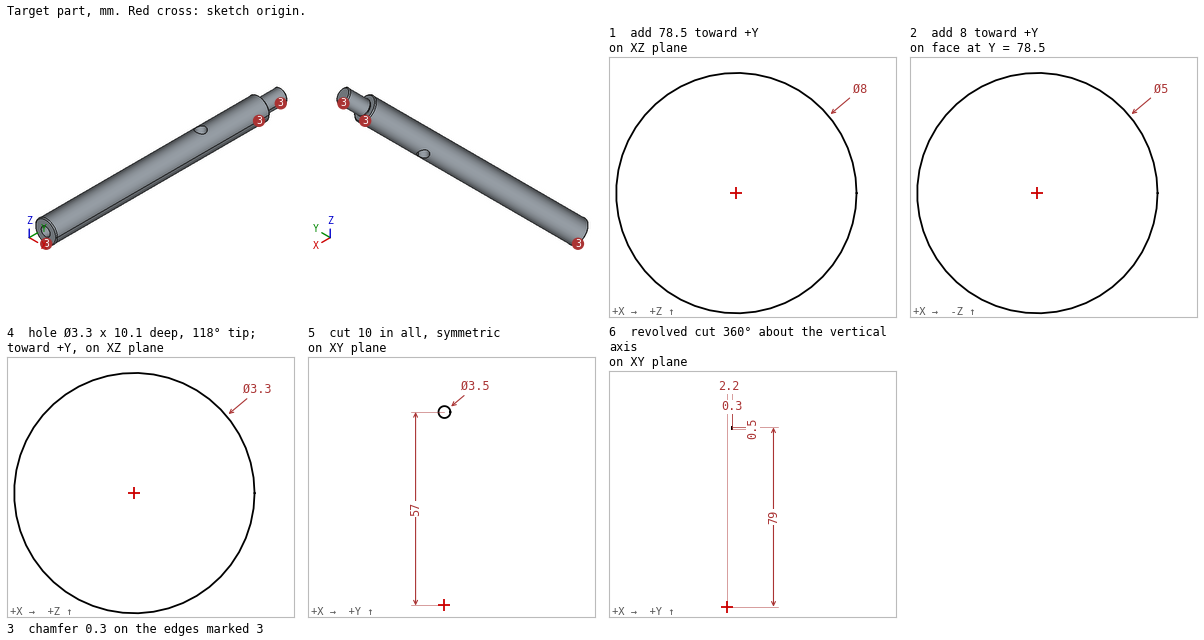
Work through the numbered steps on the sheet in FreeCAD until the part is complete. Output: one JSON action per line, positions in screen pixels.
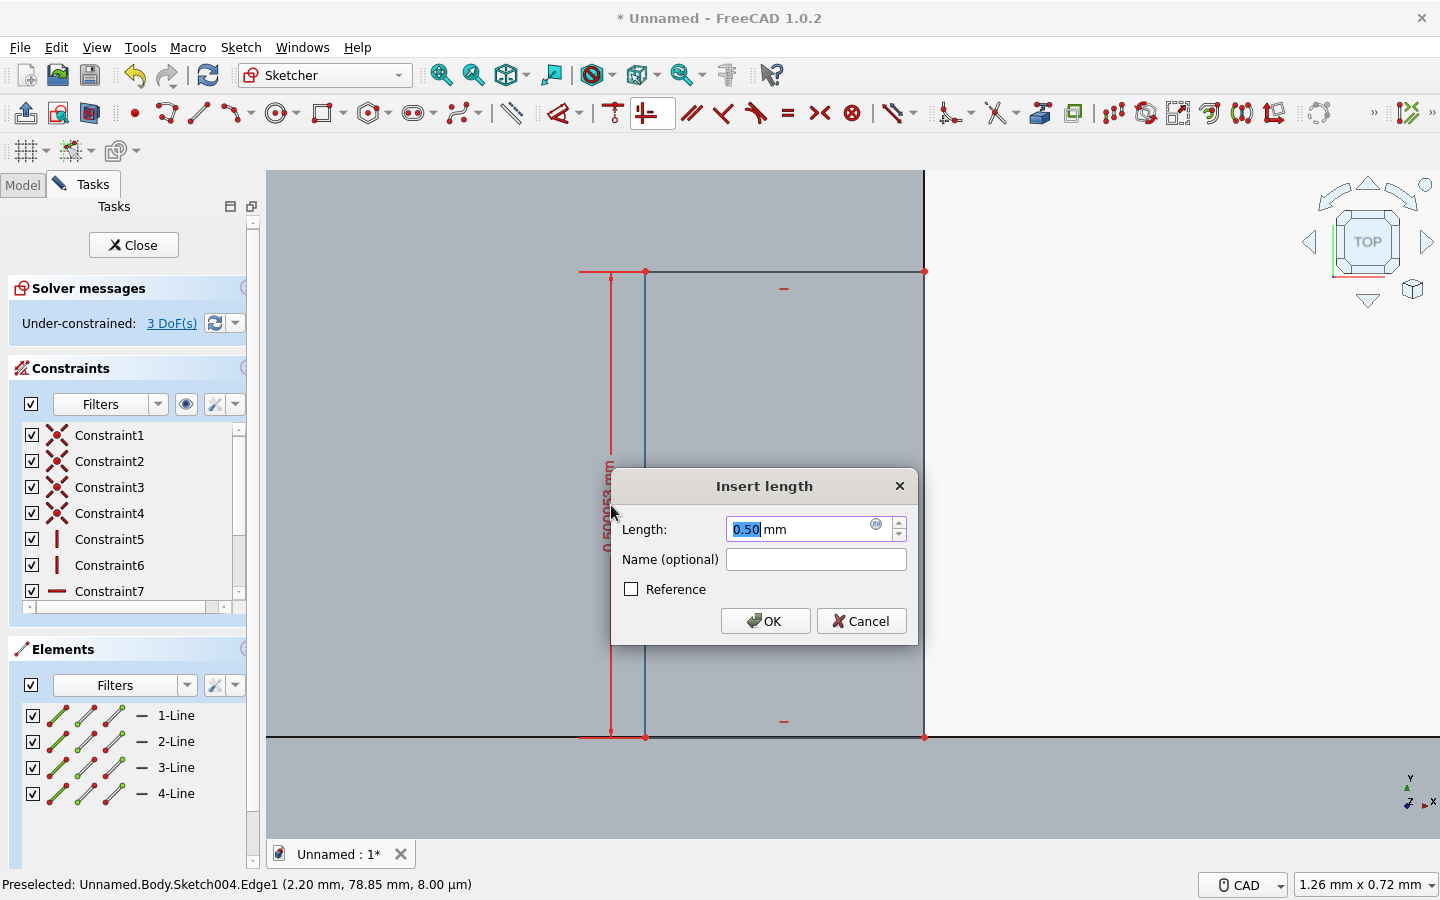
{"action": "type", "text": "0.5"}
{"action": "key", "text": "Return"}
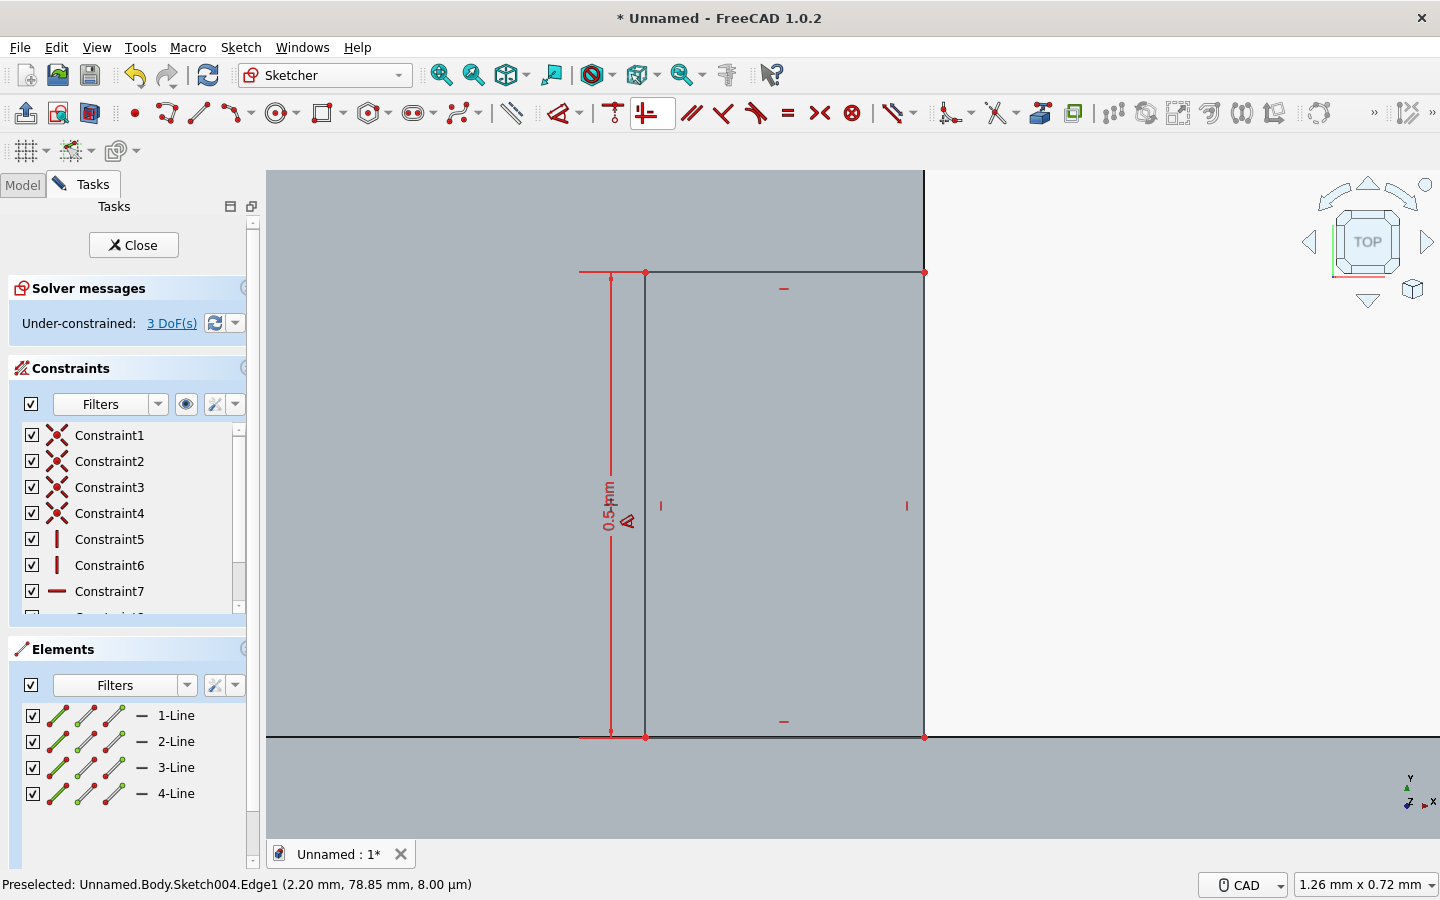
{"action": "left_click", "coordinate": [729, 738]}
{"action": "left_click", "coordinate": [785, 772]}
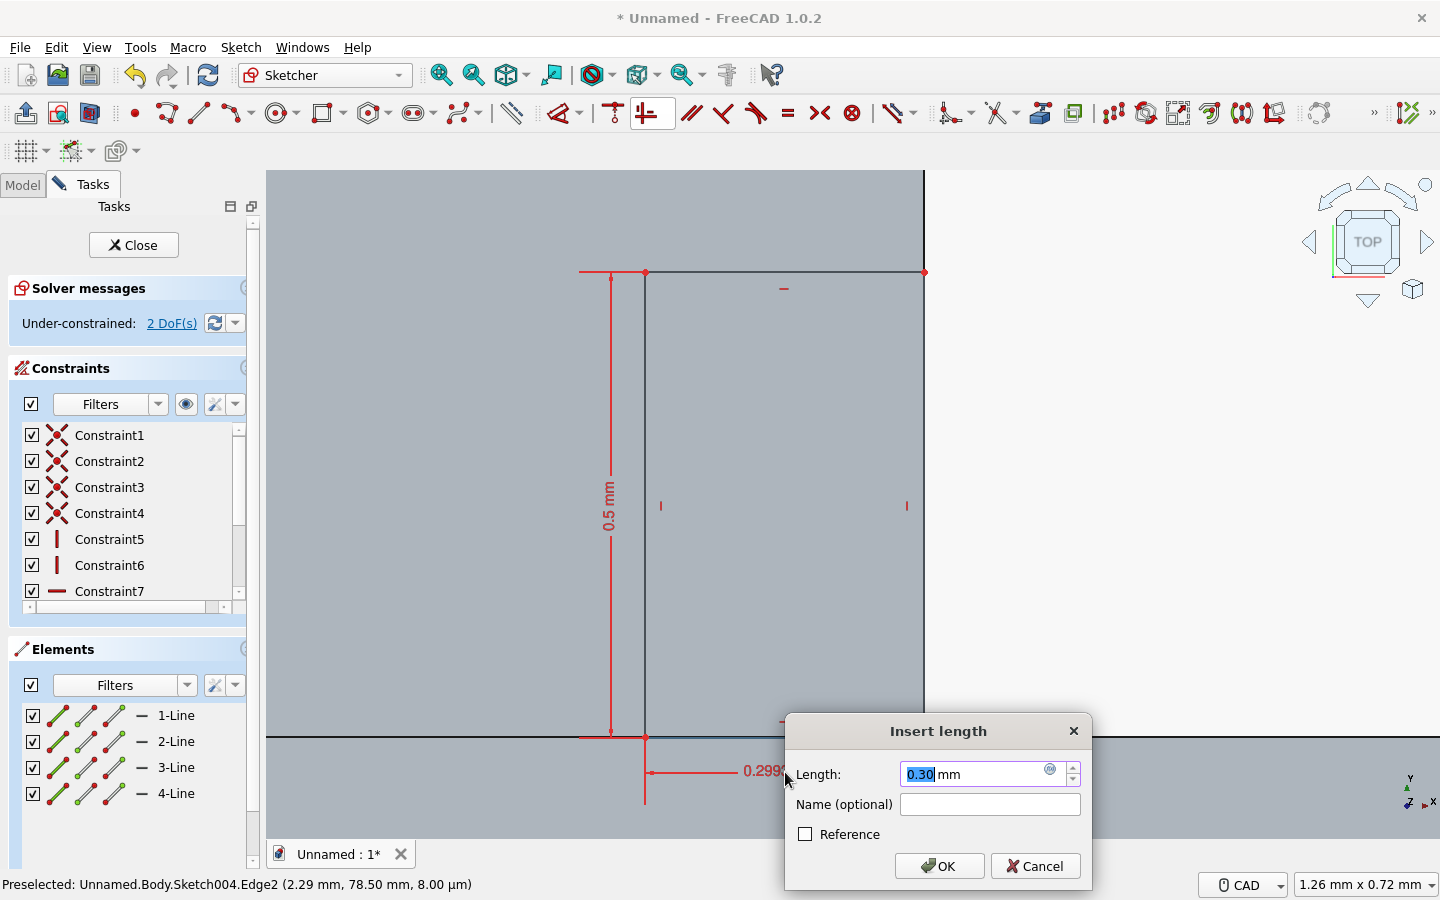
{"action": "type", "text": "0.3"}
{"action": "key", "text": "Return"}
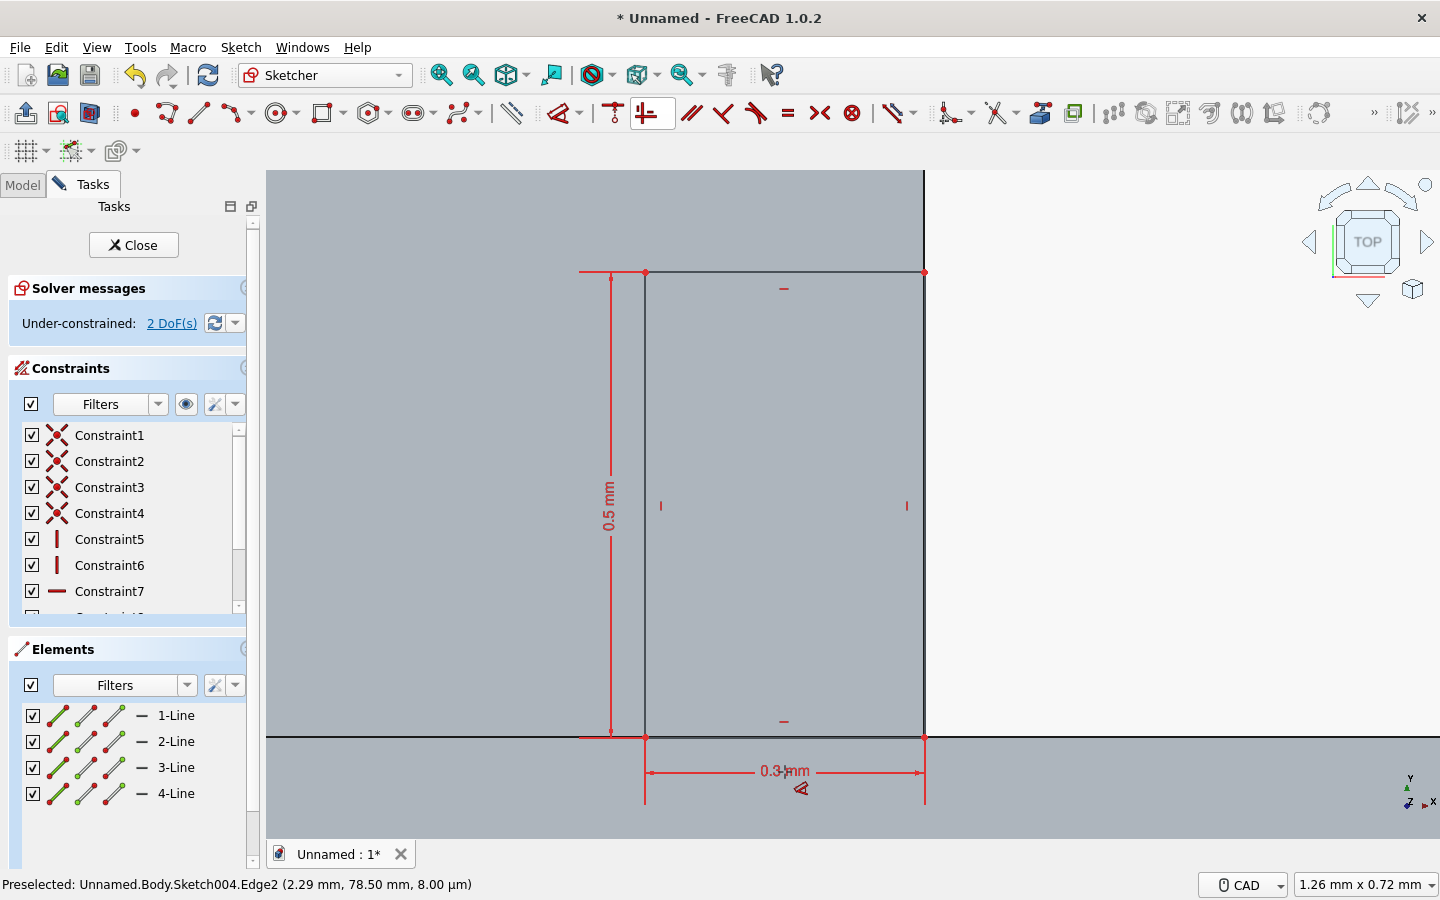
{"action": "left_click", "coordinate": [645, 272]}
{"action": "left_click", "coordinate": [679, 542]}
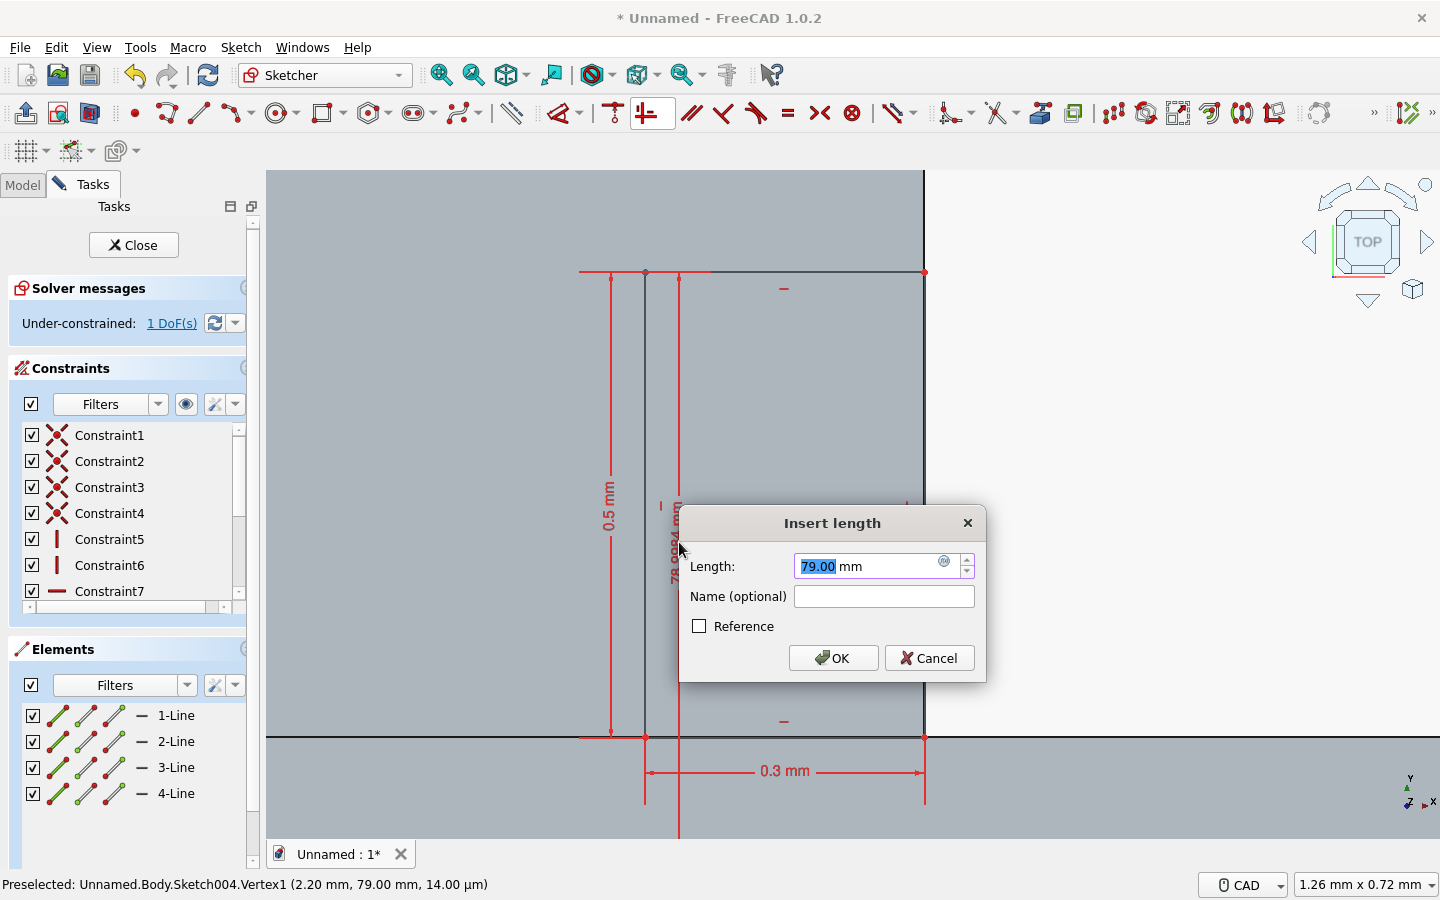
{"action": "type", "text": "79"}
{"action": "key", "text": "Return"}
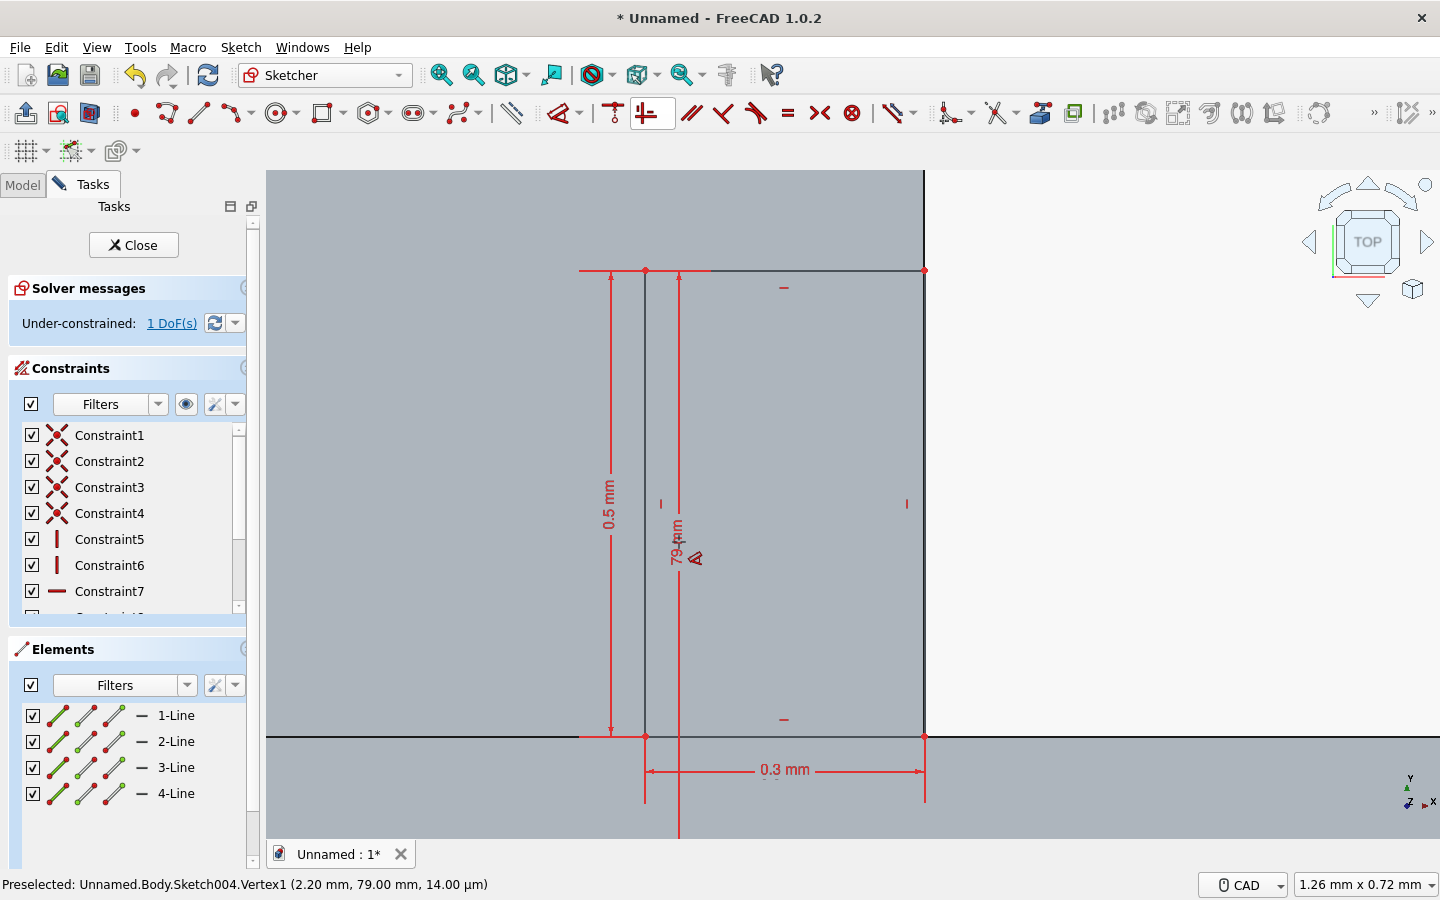
{"action": "left_click", "coordinate": [645, 271]}
{"action": "left_click", "coordinate": [470, 237]}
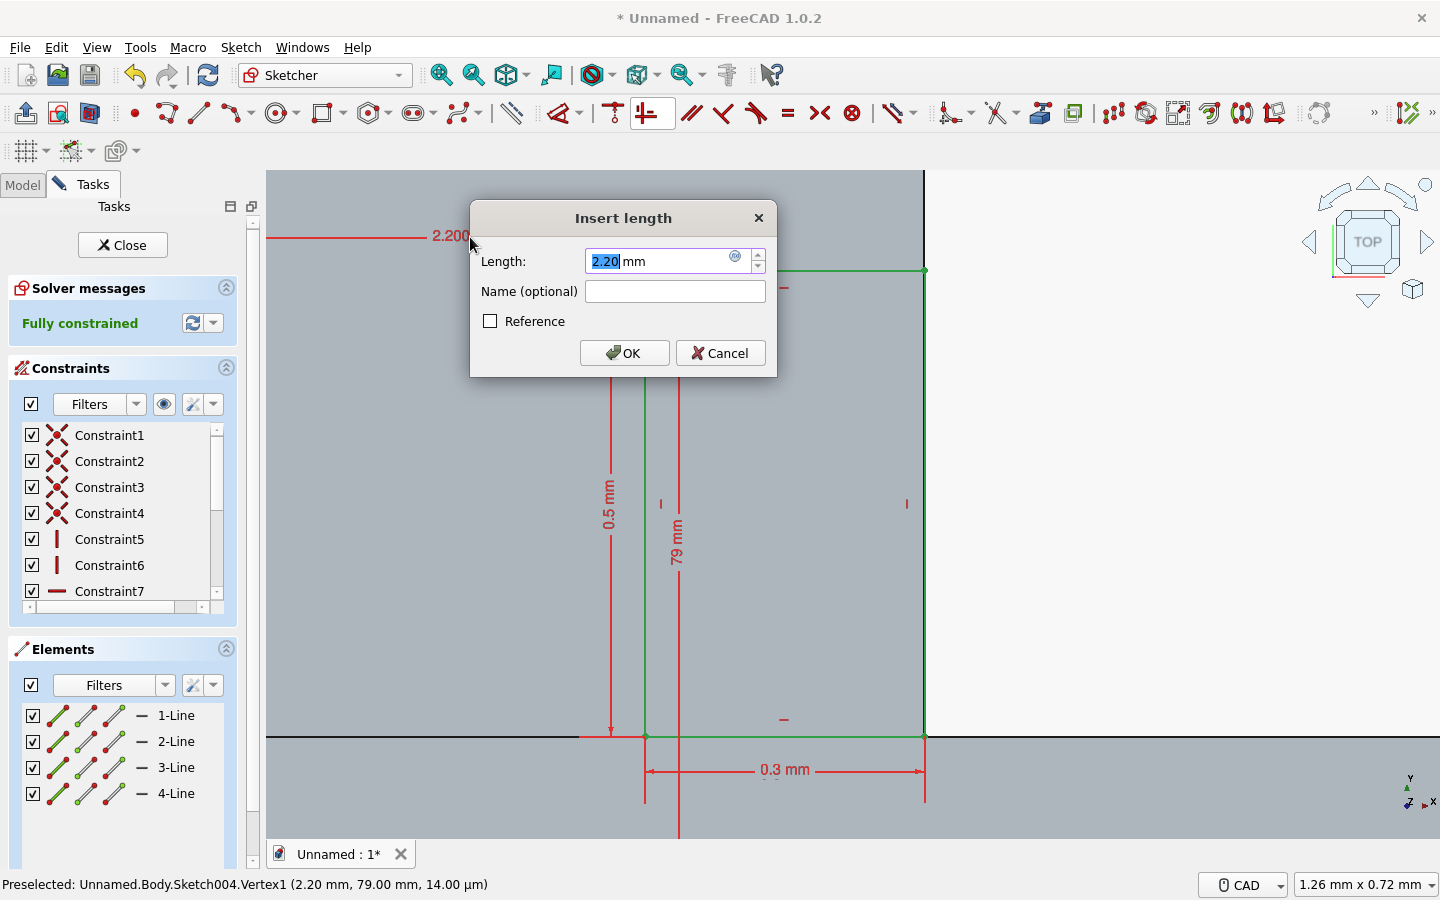
{"action": "type", "text": "2.2"}
{"action": "key", "text": "Return"}
{"action": "key", "text": "Escape"}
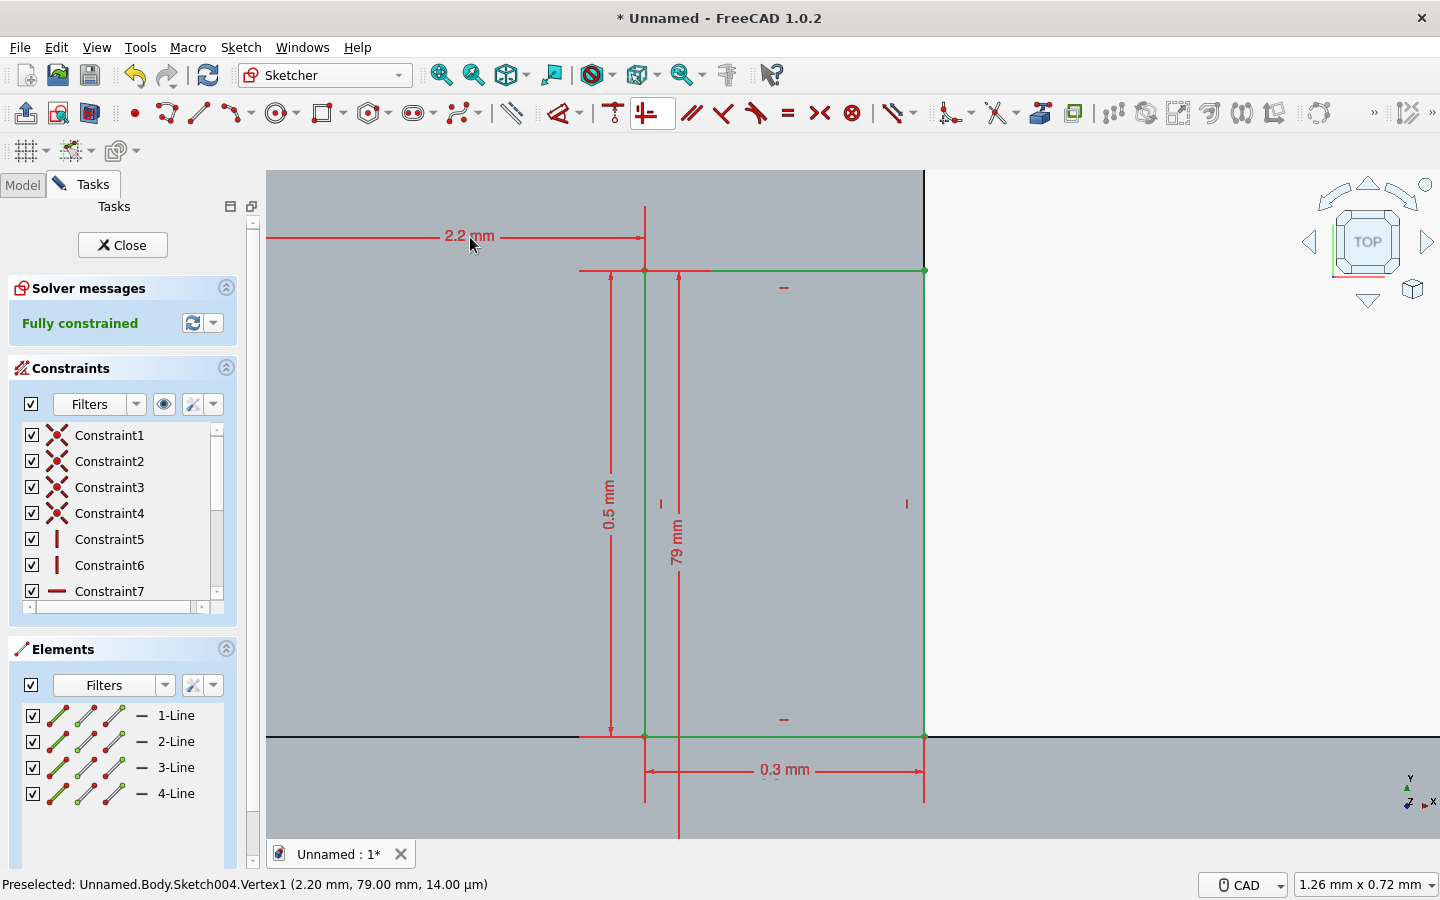
{"action": "left_click", "coordinate": [123, 245]}